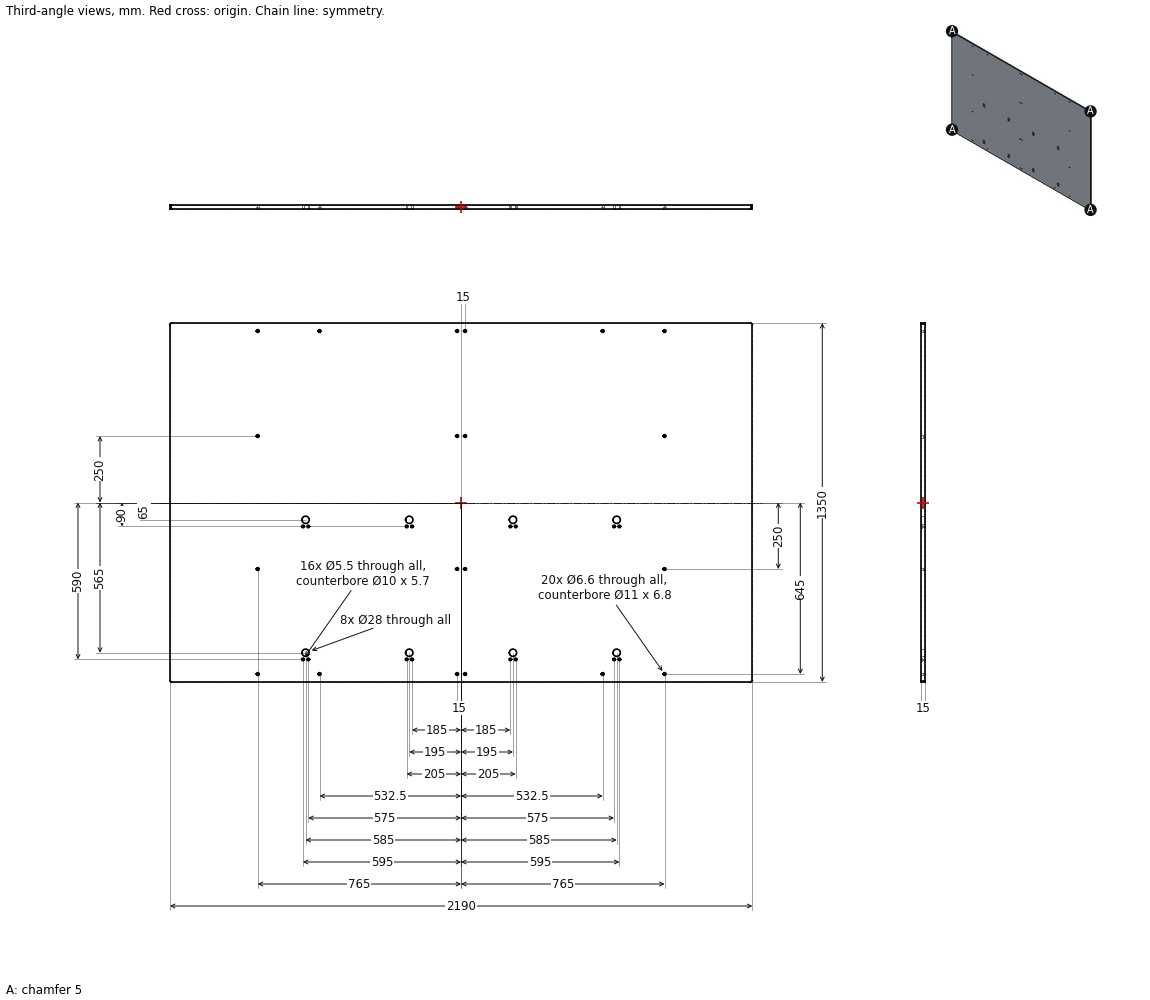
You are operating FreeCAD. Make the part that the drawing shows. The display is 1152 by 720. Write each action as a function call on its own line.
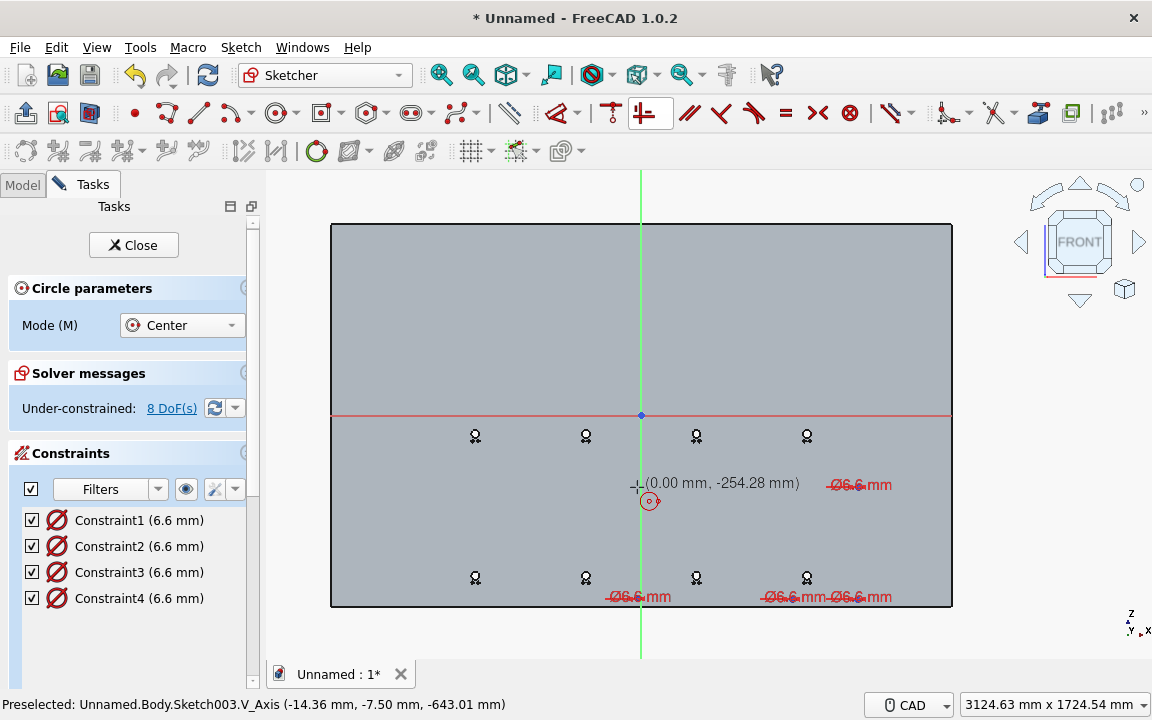
scroll(637, 486, up, 7)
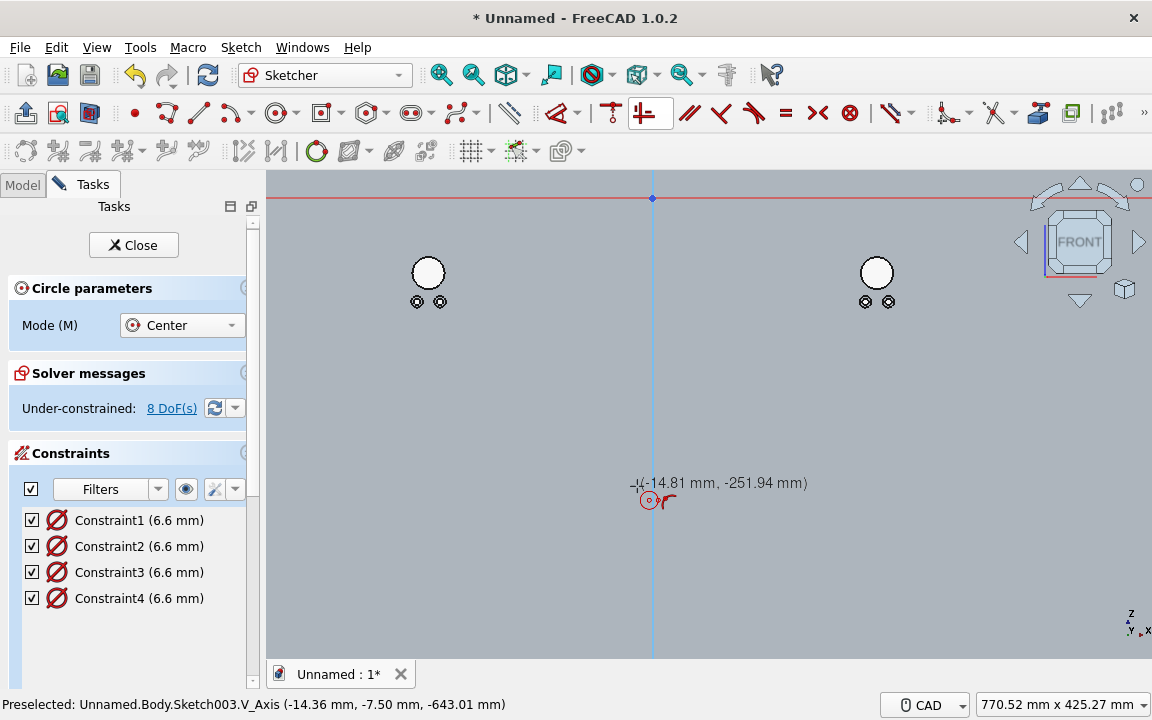
click(636, 486)
move(638, 483)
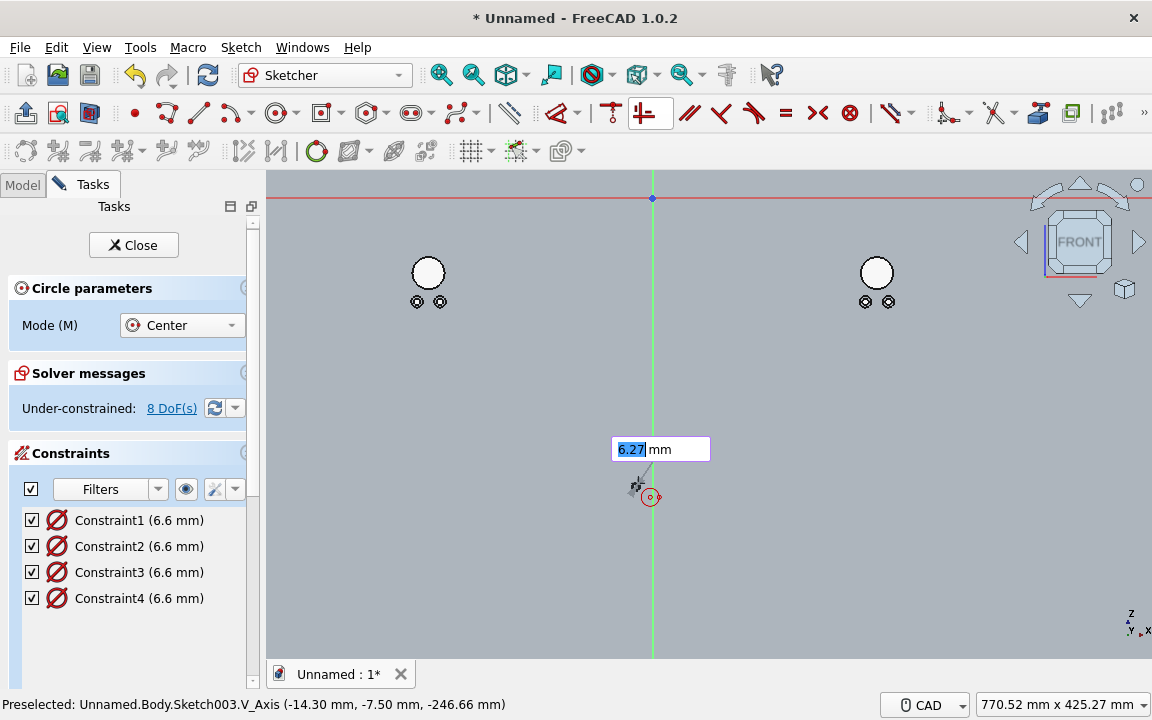
text(6.6)
key(Return)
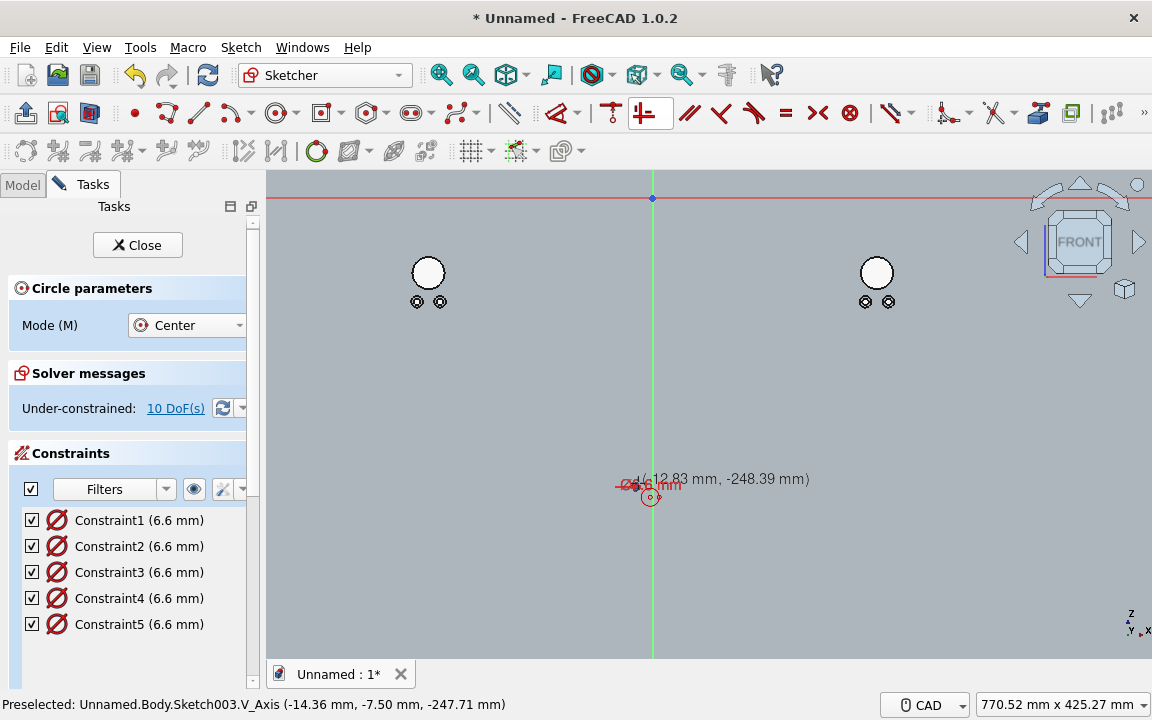
scroll(637, 469, down, 8)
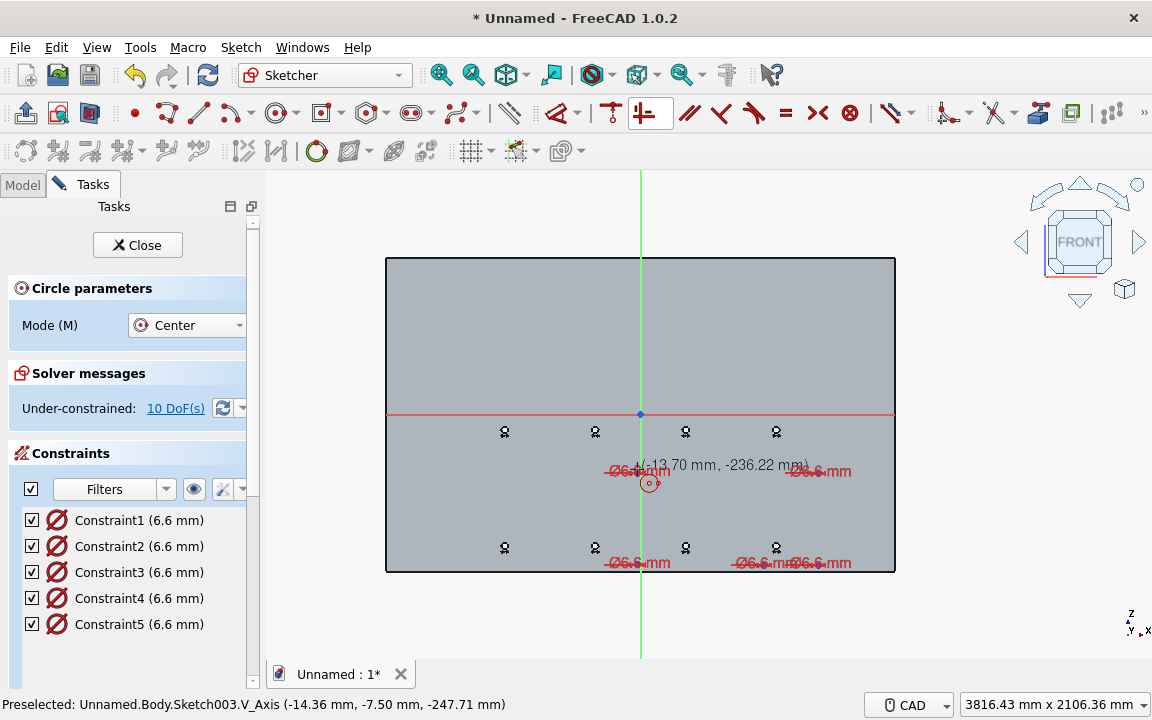
scroll(463, 473, up, 17)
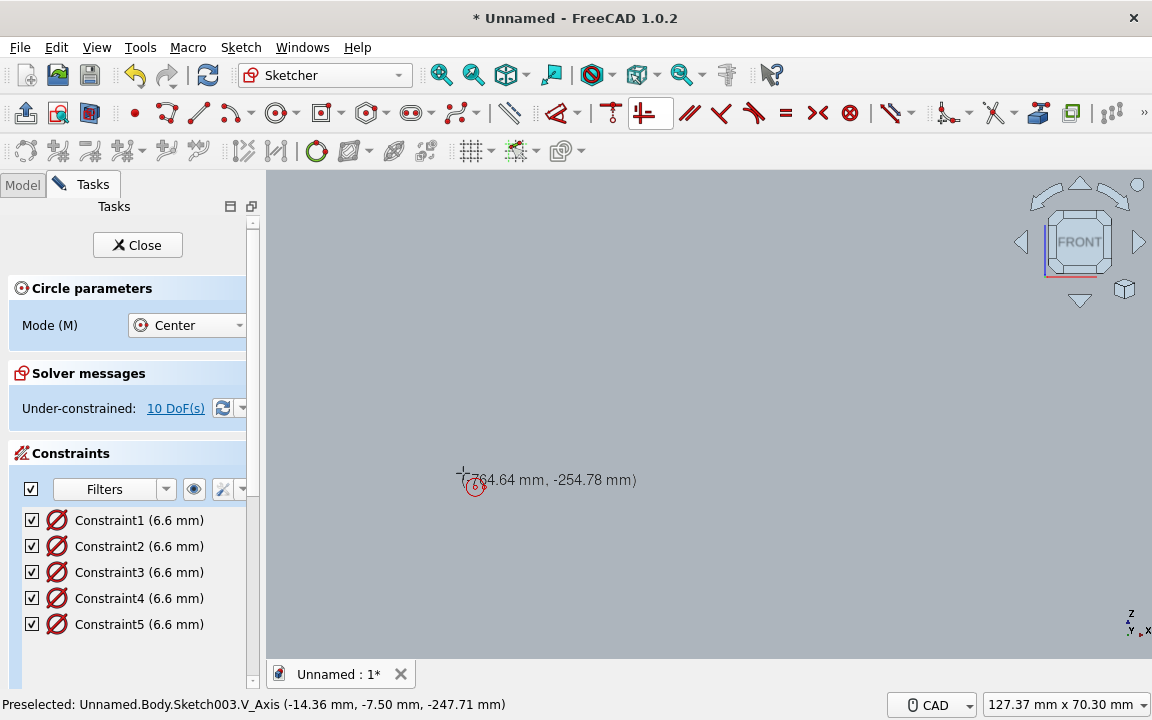
scroll(422, 487, down, 16)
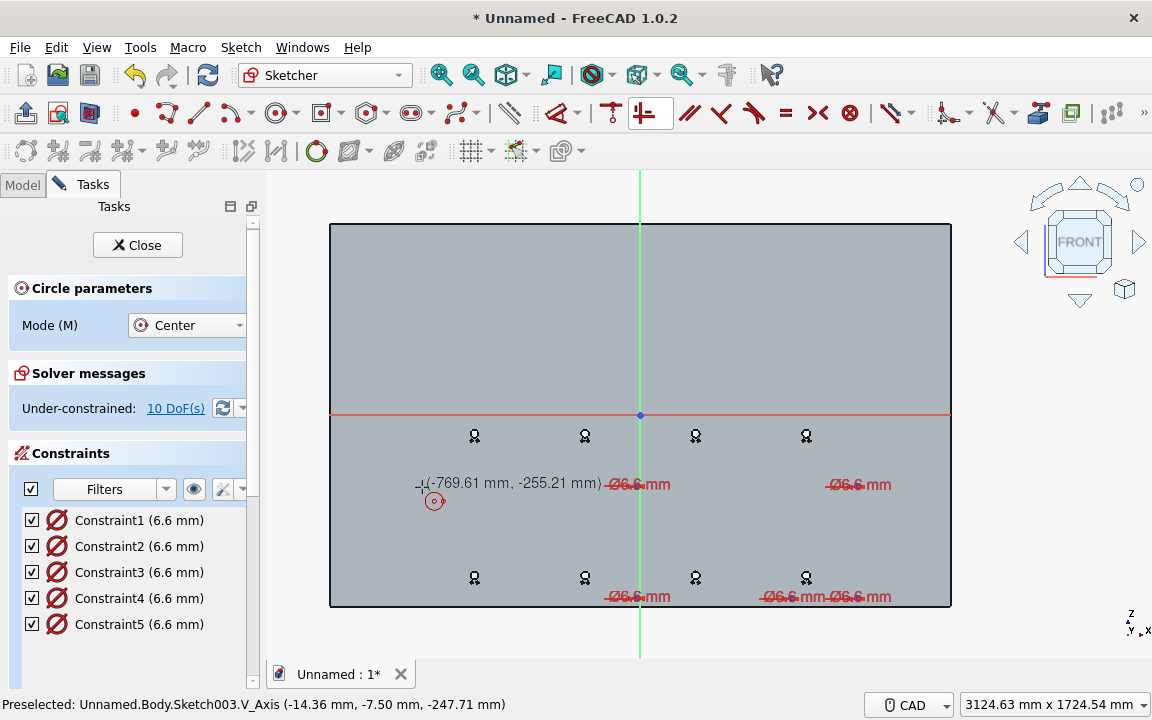
click(423, 486)
move(424, 486)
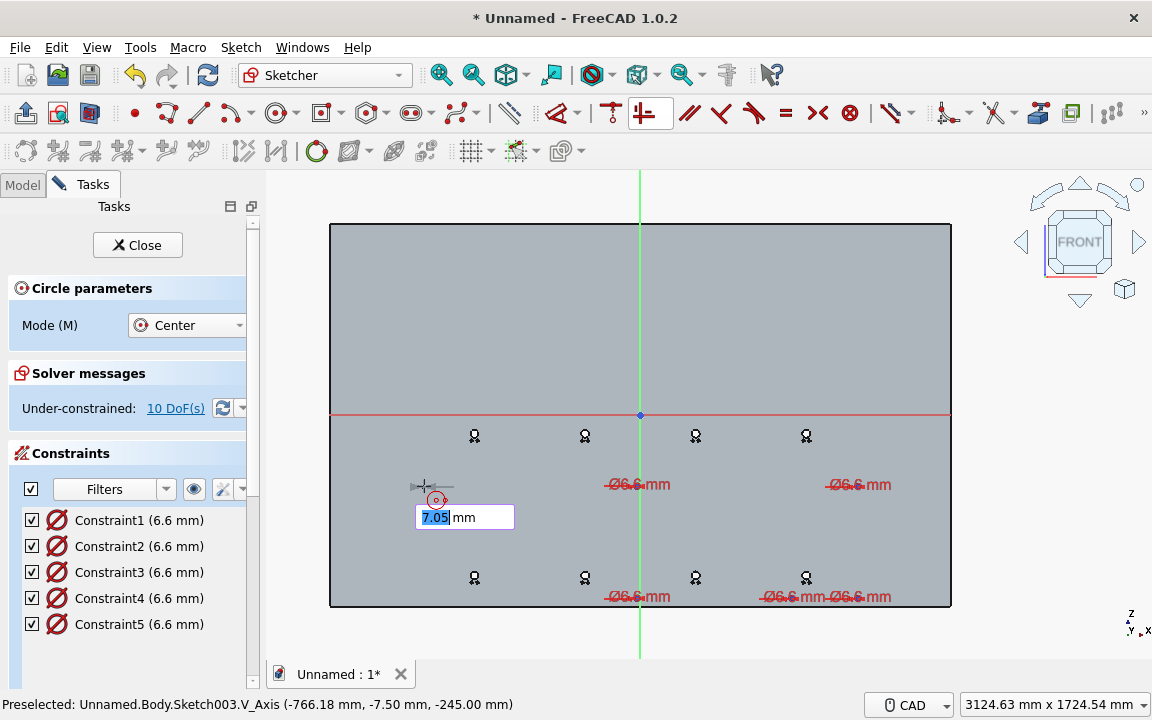
text(6.6)
key(Return)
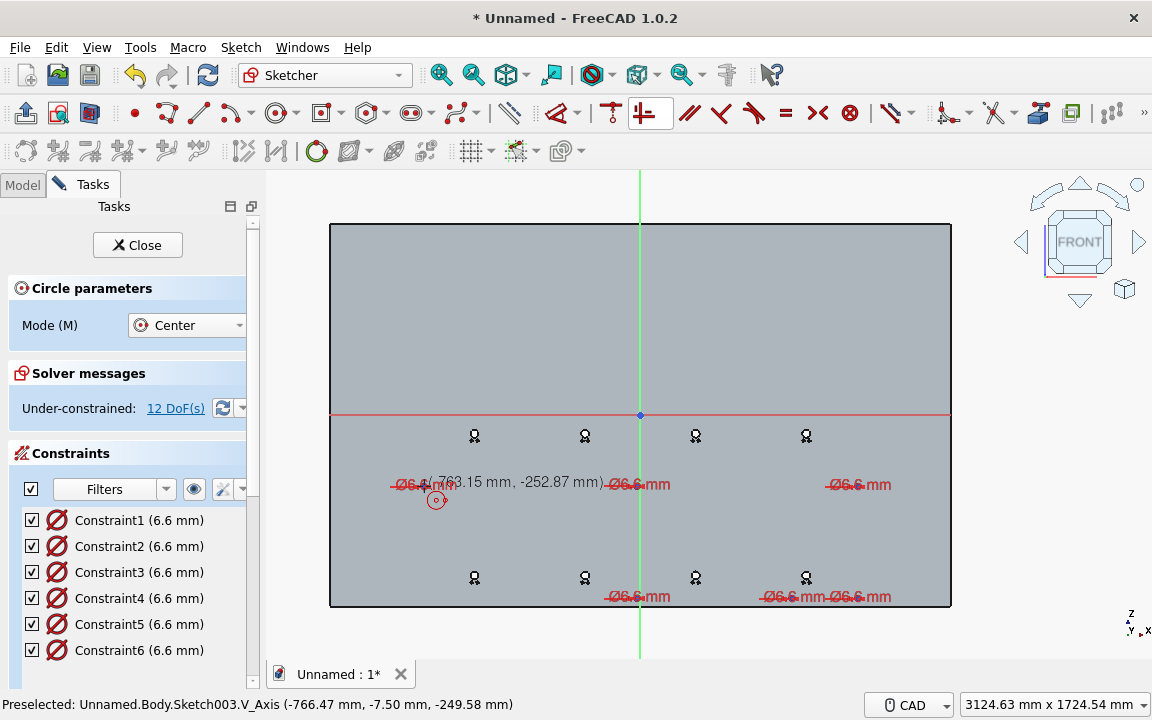
scroll(489, 598, up, 16)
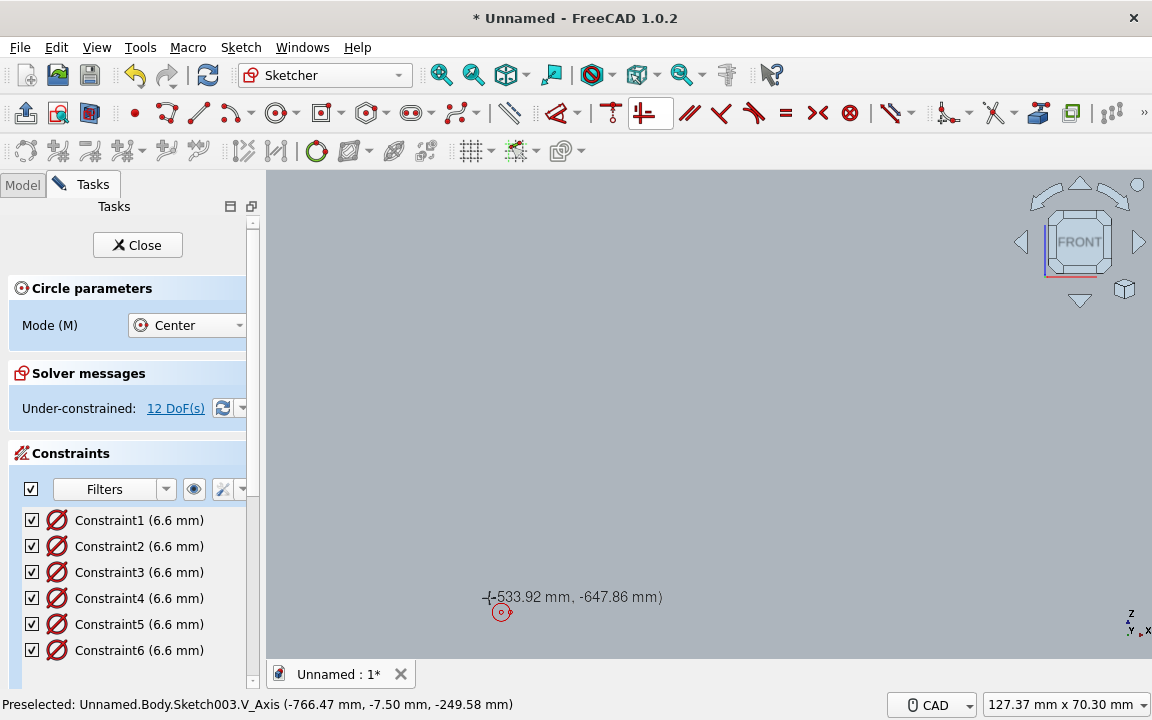
scroll(489, 598, down, 16)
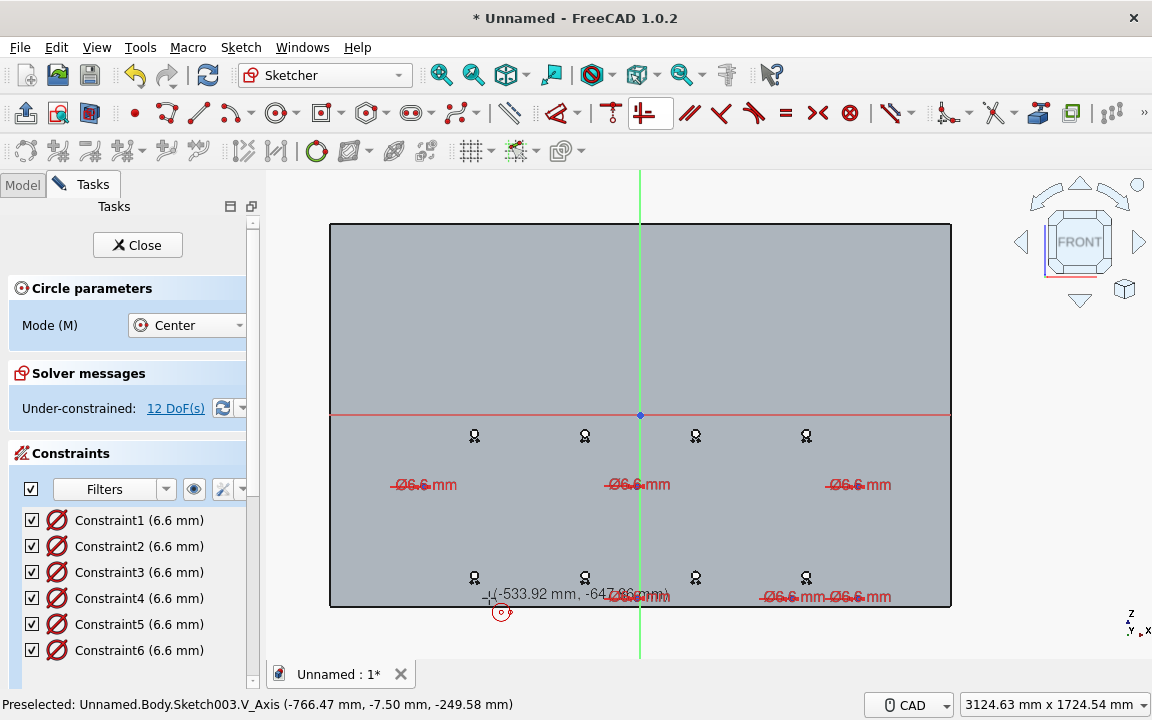
click(489, 598)
move(490, 598)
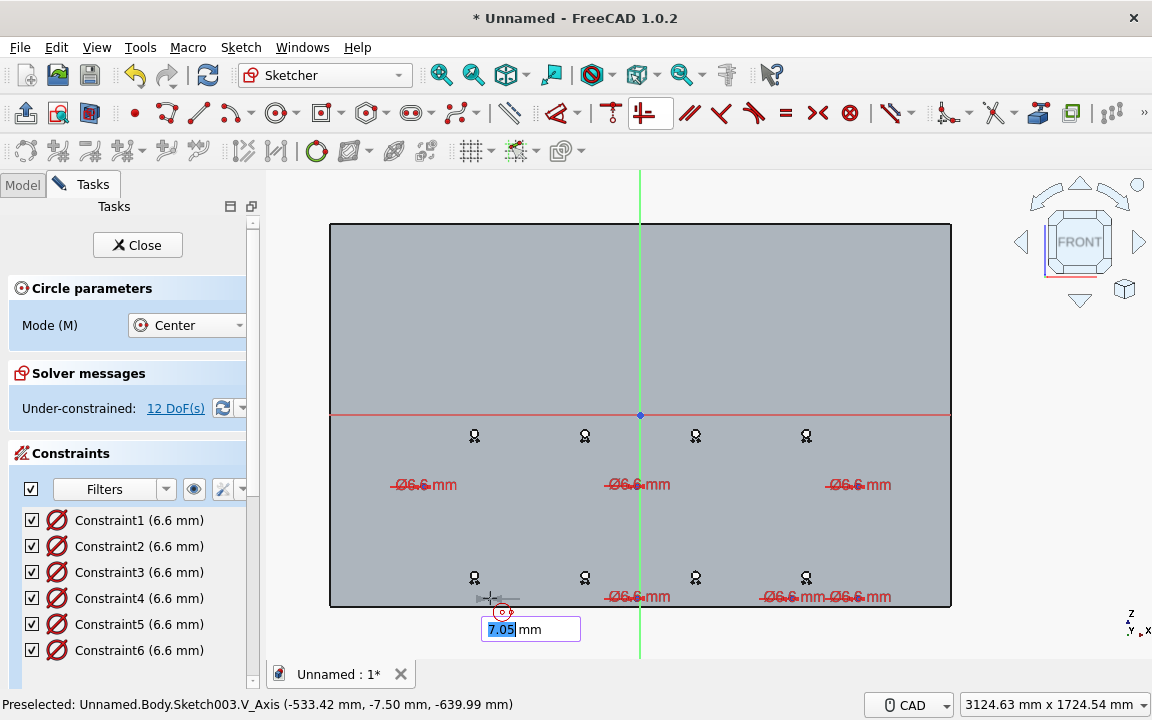
text(6.6)
key(Return)